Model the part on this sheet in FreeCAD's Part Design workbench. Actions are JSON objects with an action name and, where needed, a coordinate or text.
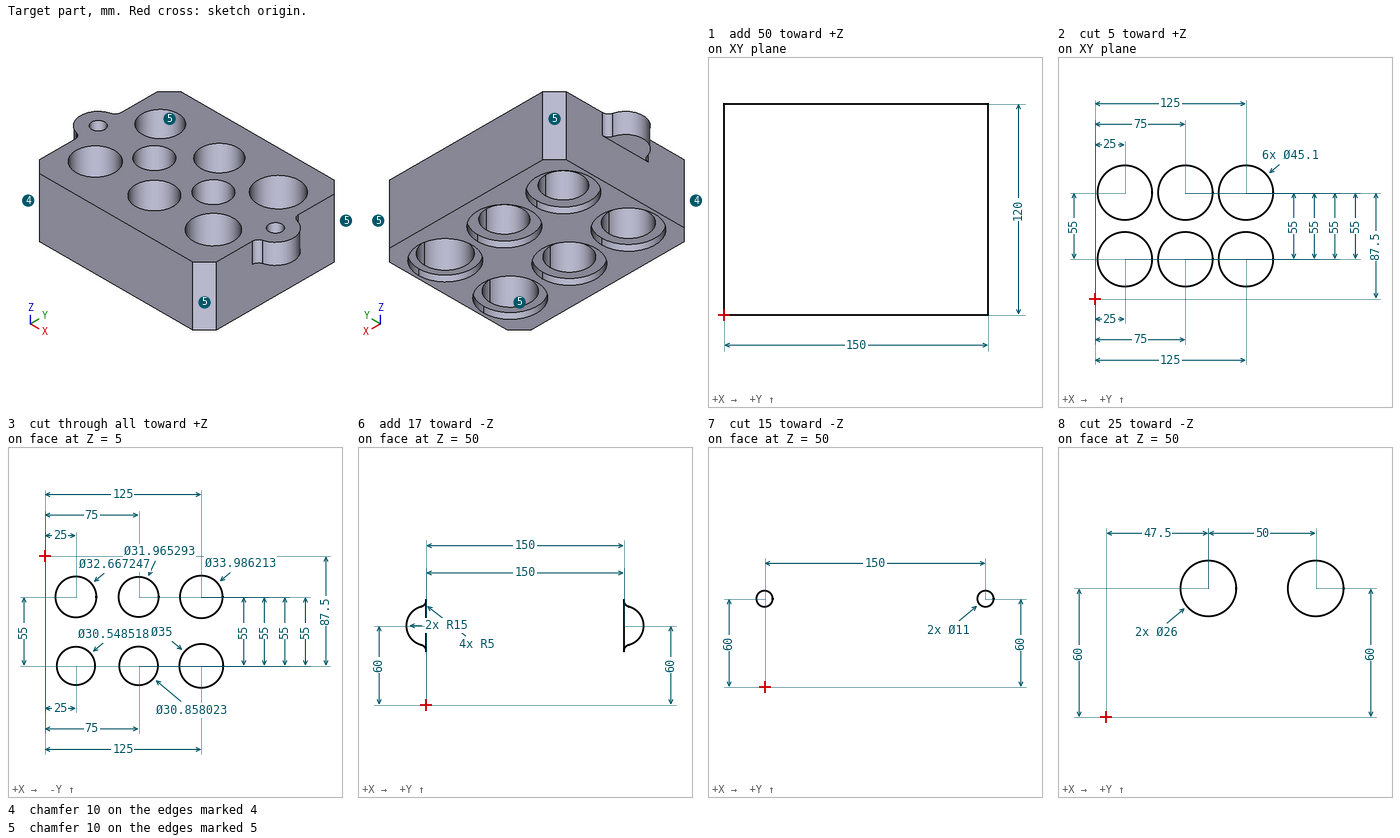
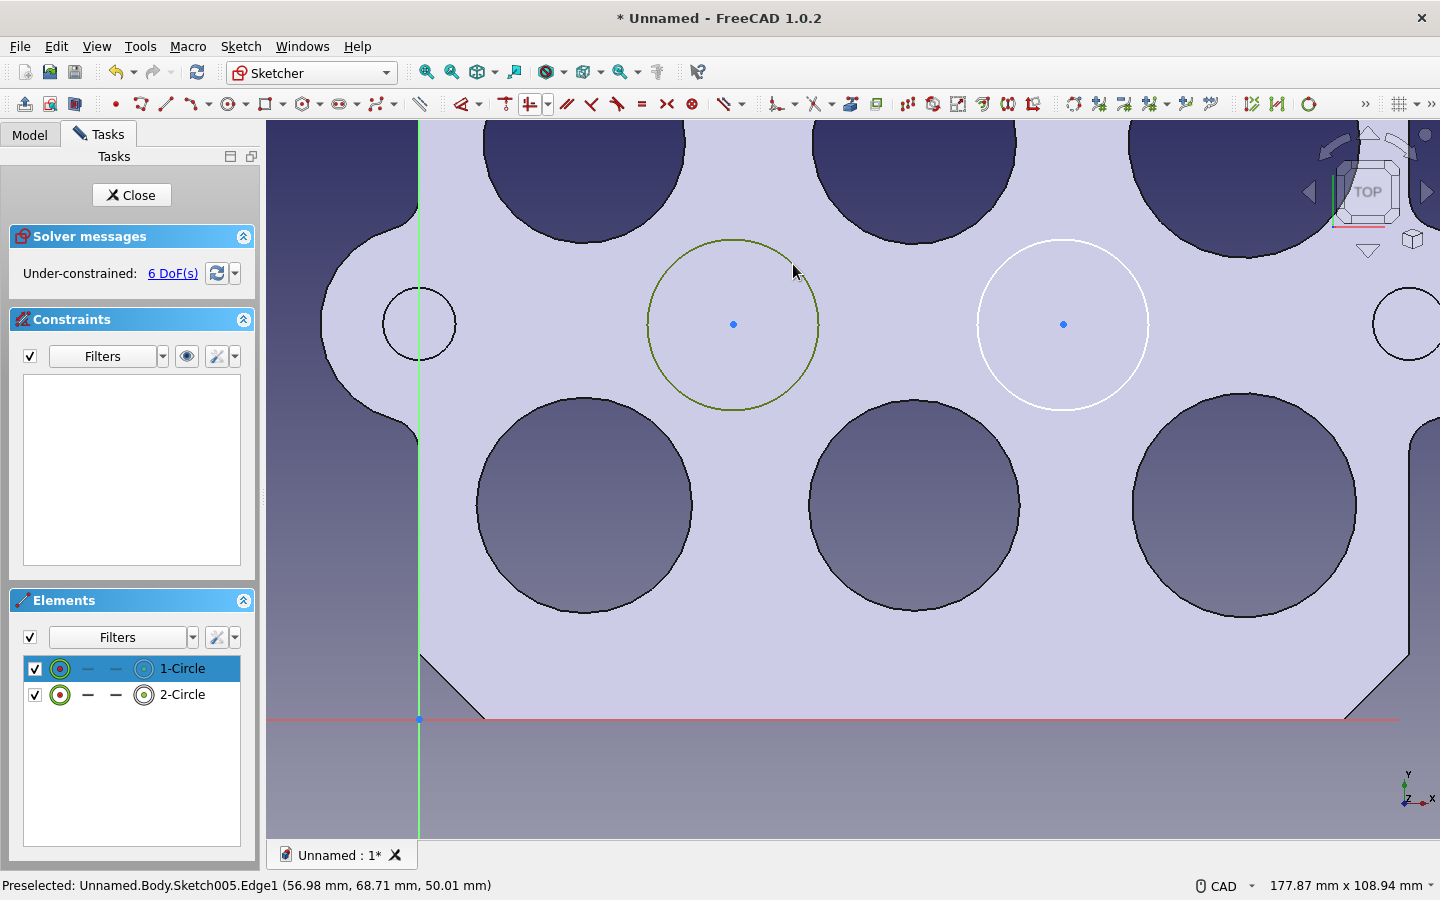
{"action": "left_click", "coordinate": [1123, 264]}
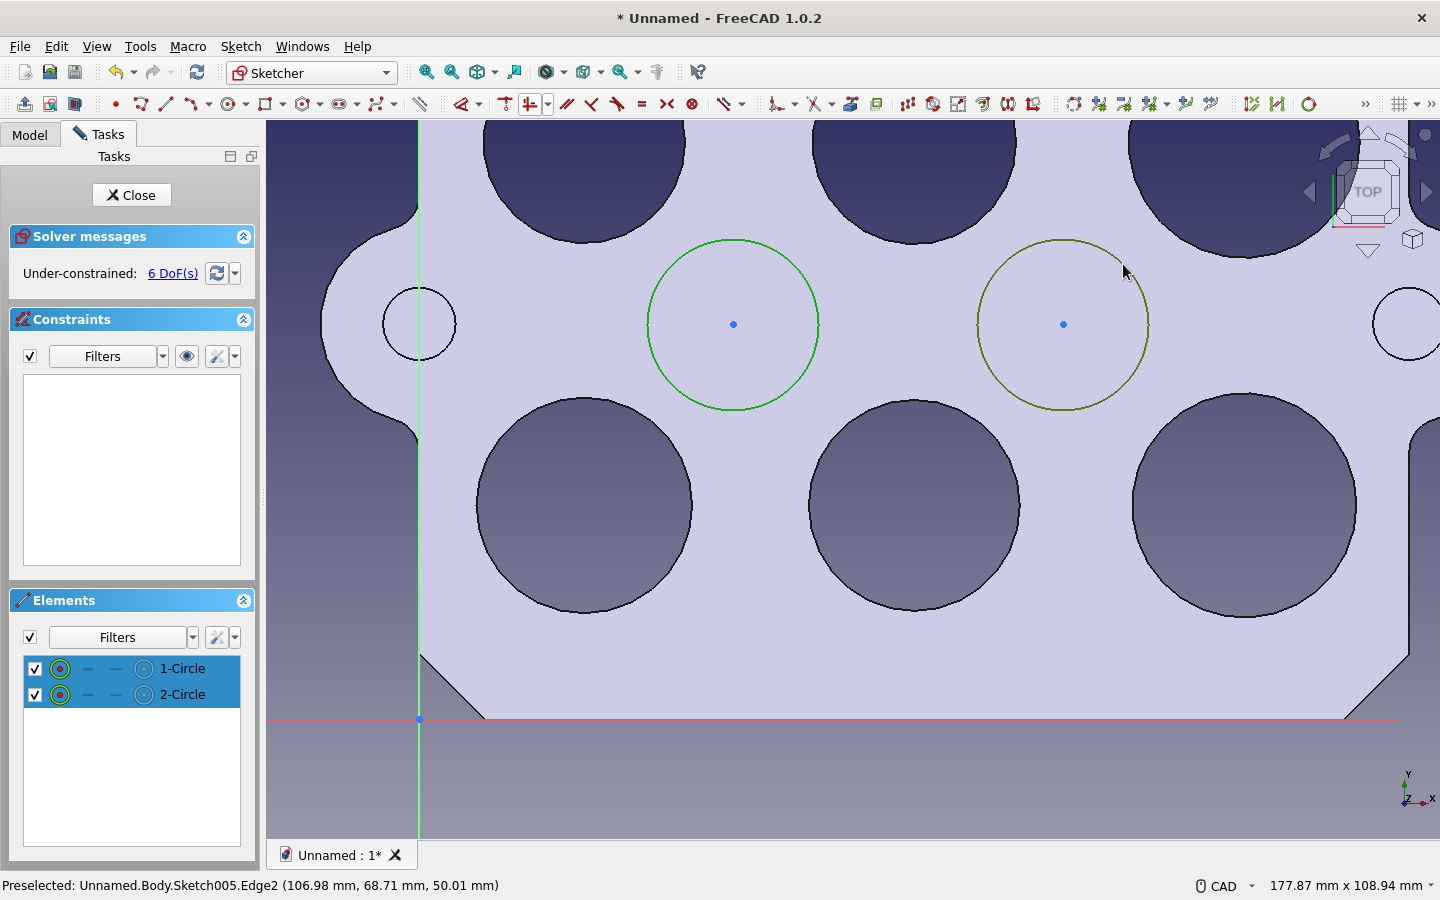
{"action": "left_click", "coordinate": [642, 104]}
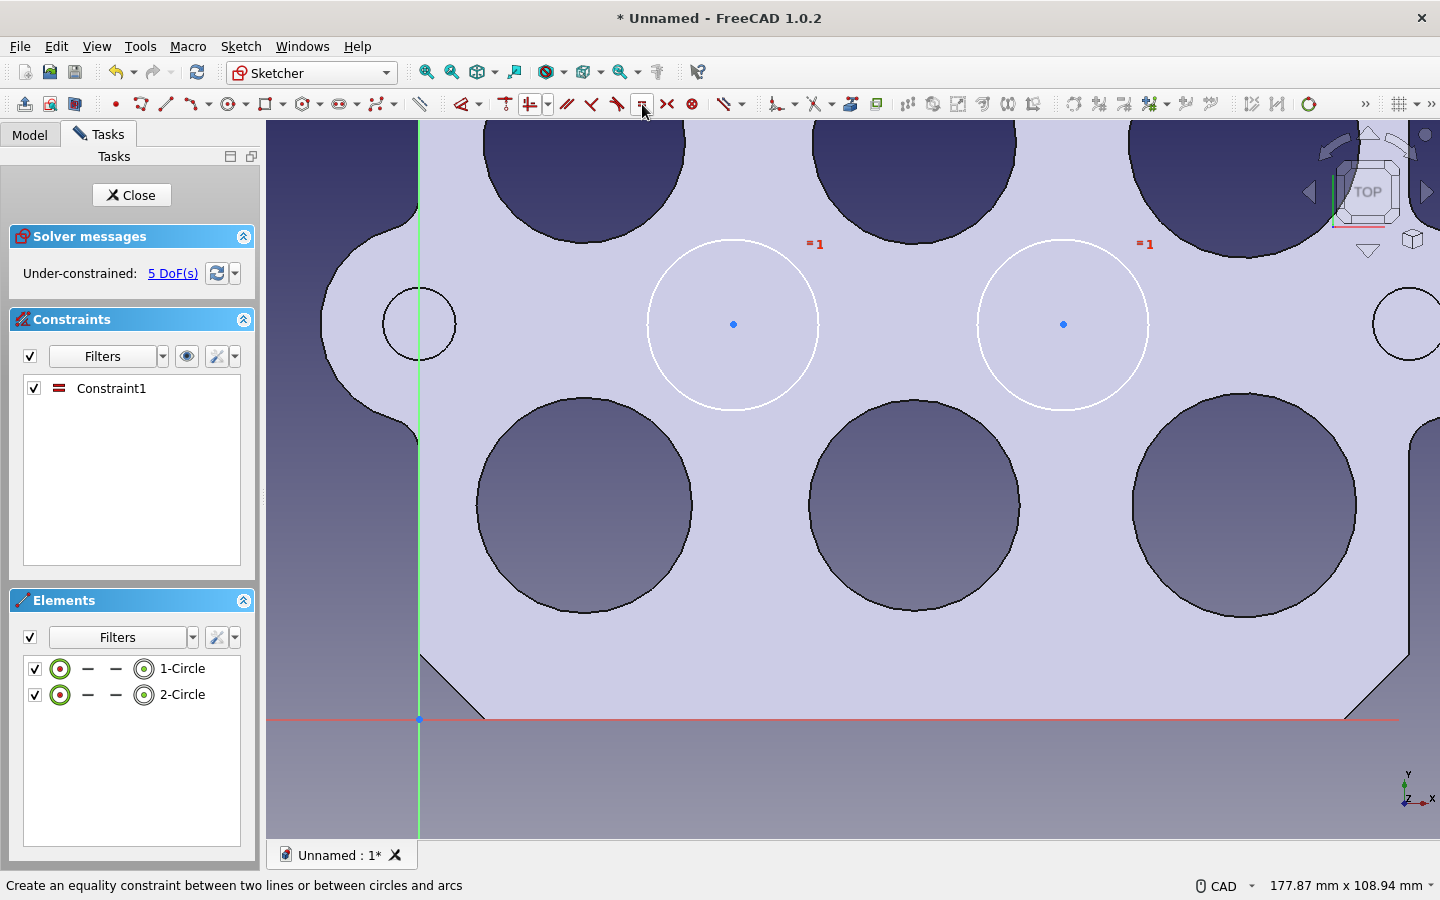
{"action": "left_click", "coordinate": [460, 104]}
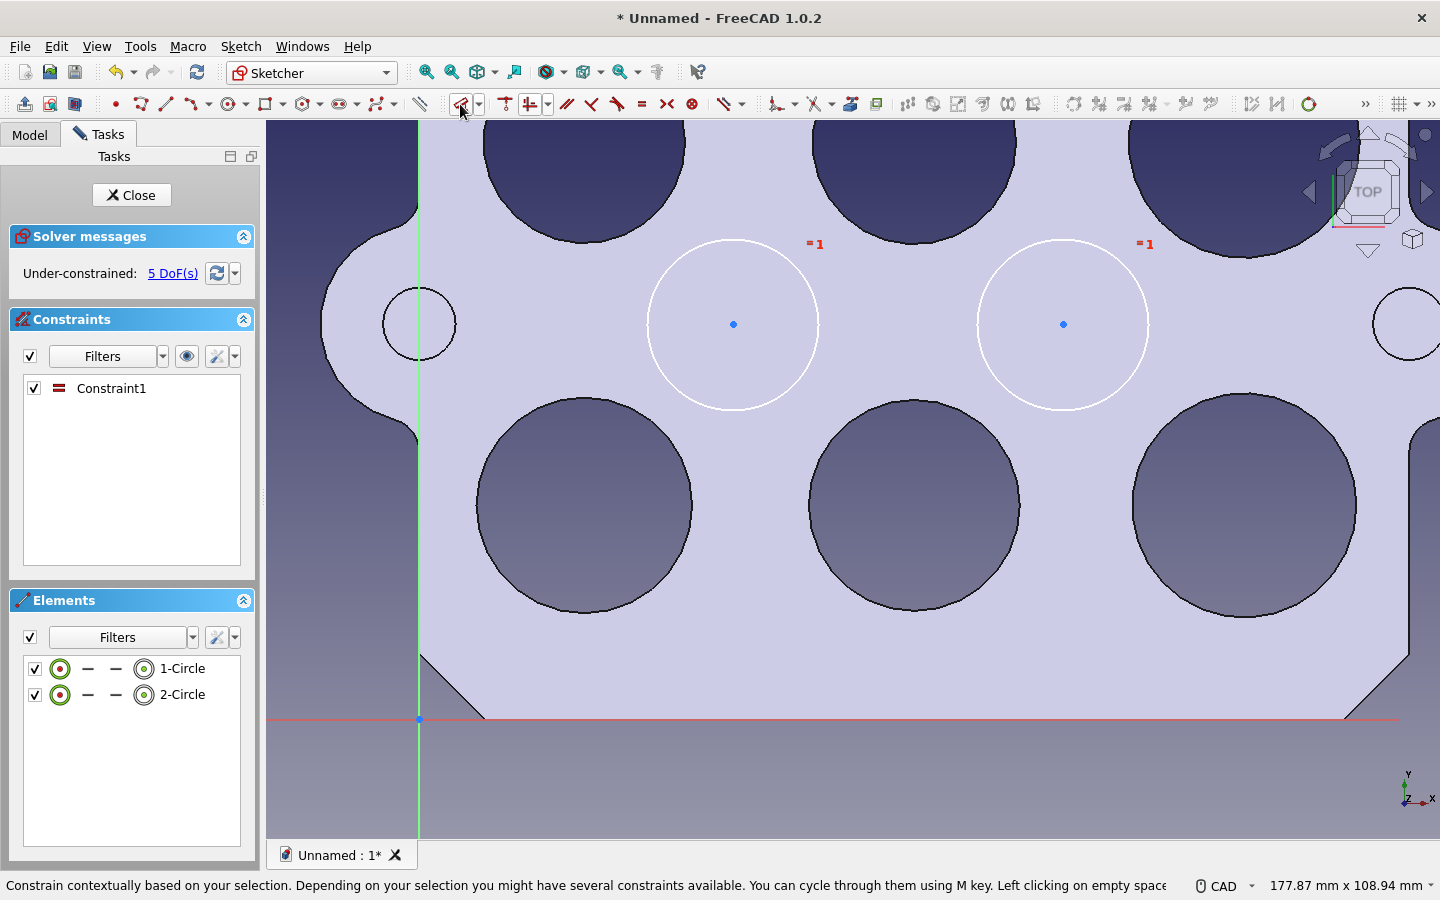
{"action": "left_click", "coordinate": [793, 264]}
{"action": "left_click", "coordinate": [815, 241]}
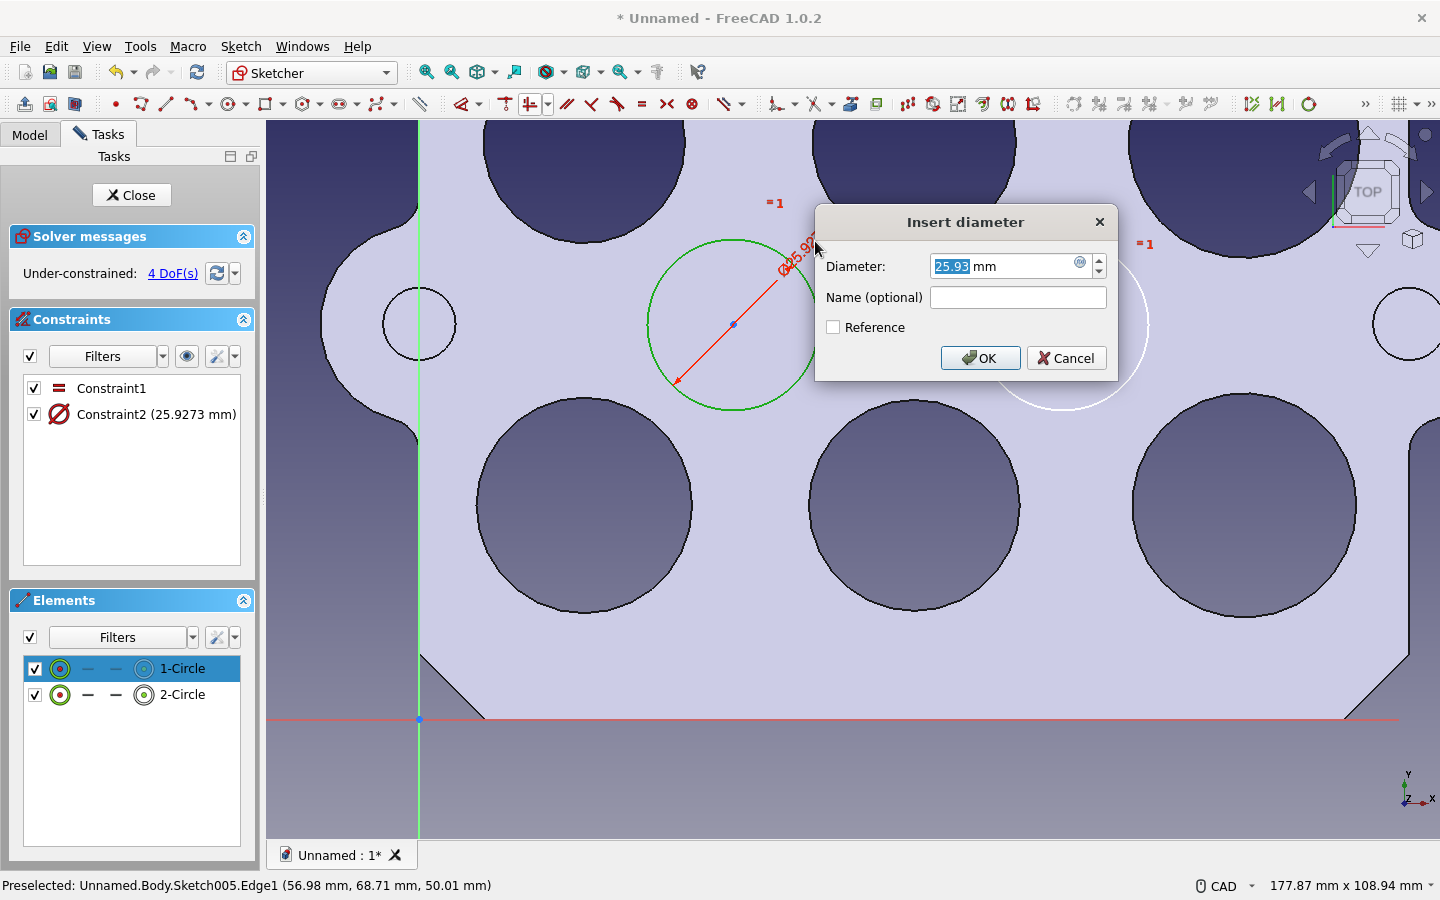
{"action": "type", "text": "26"}
{"action": "key", "text": "Return"}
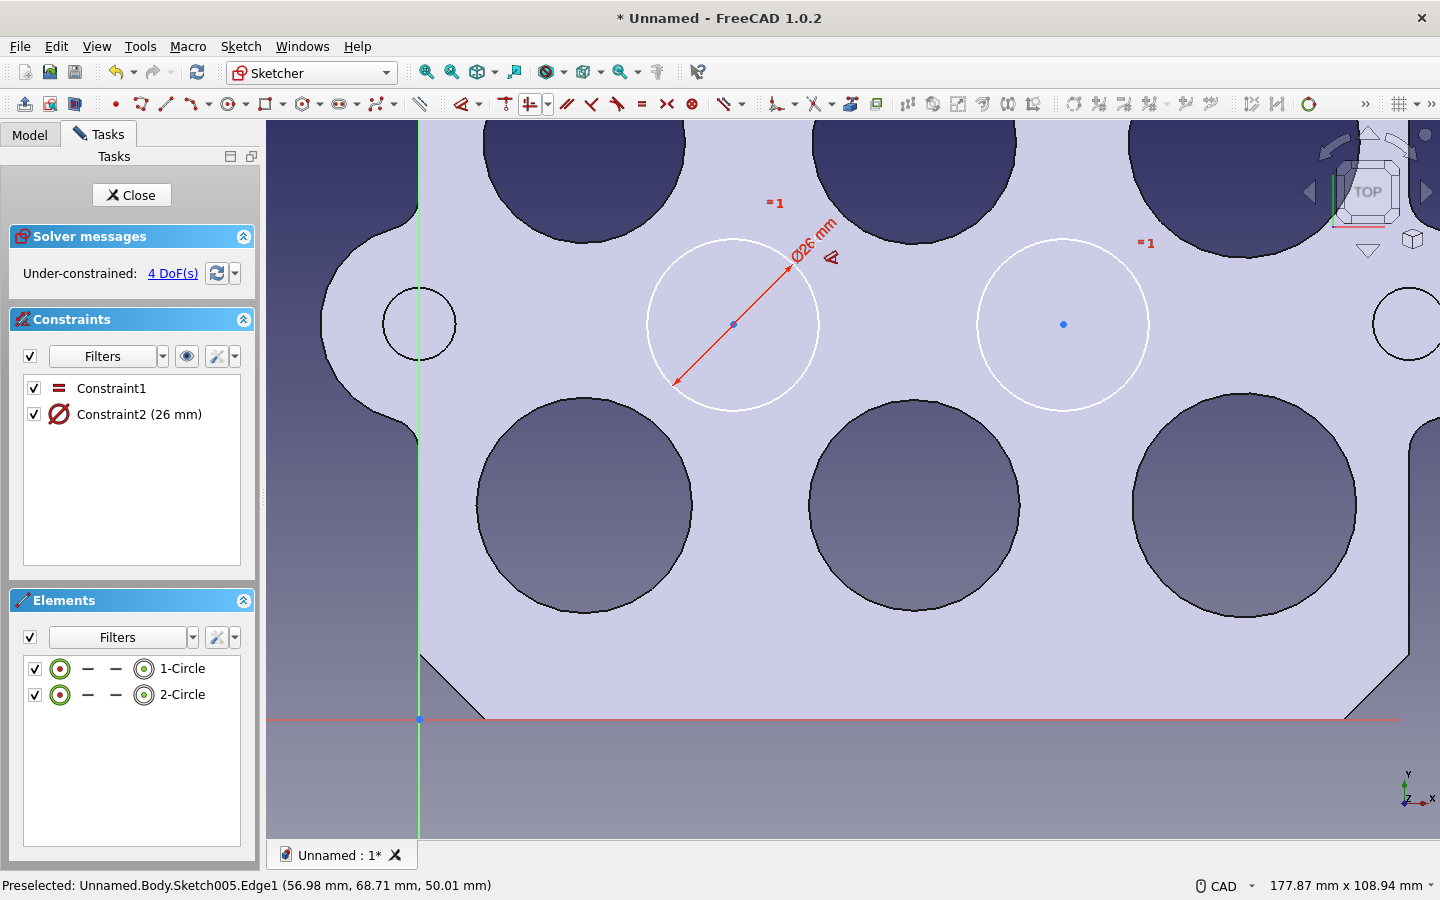
{"action": "left_click", "coordinate": [733, 325]}
{"action": "left_click", "coordinate": [385, 522]}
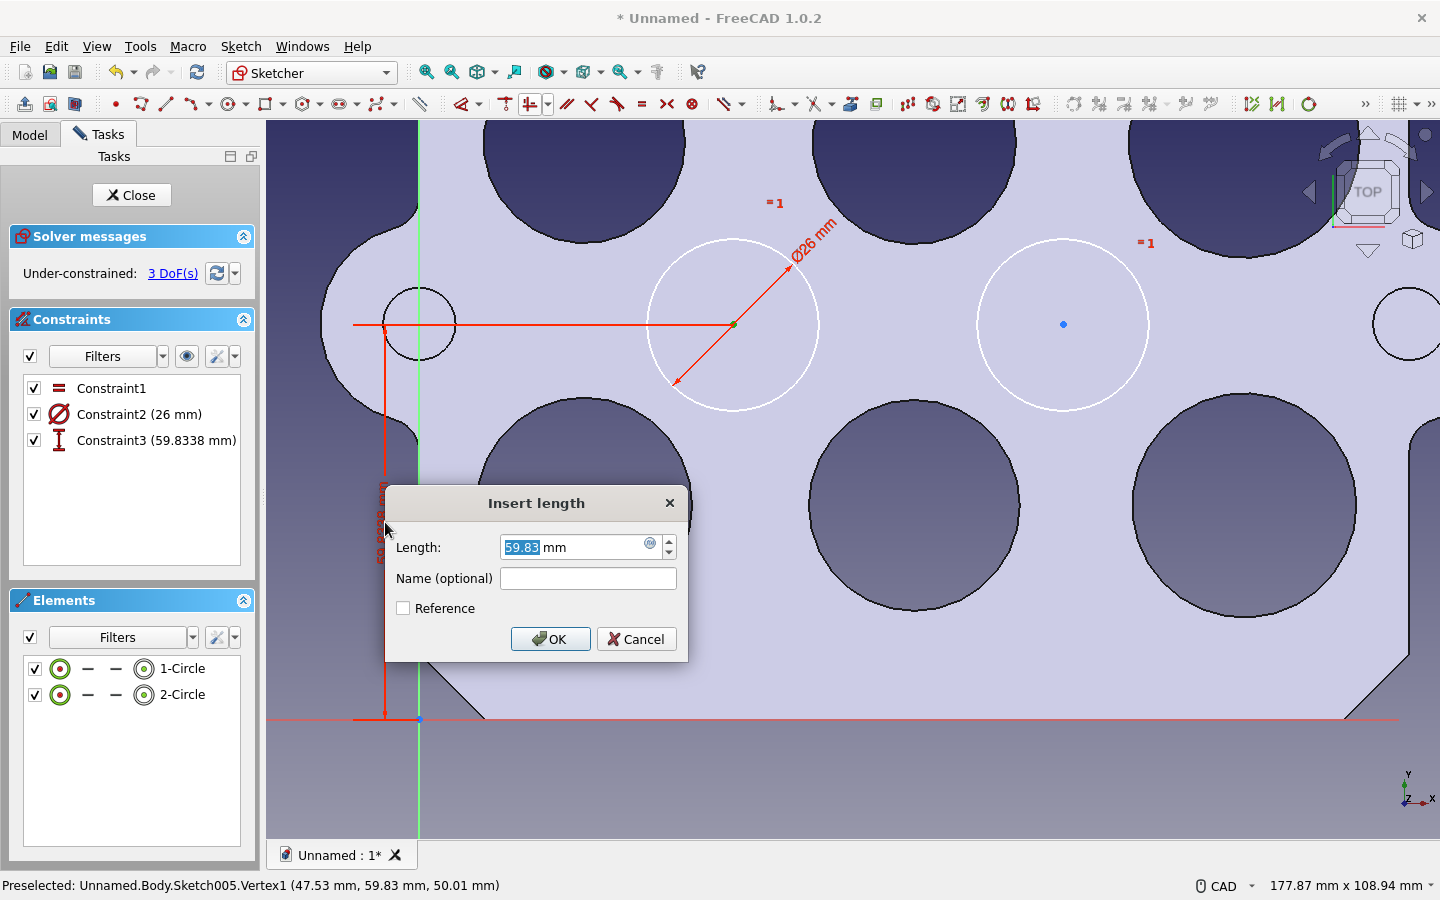
{"action": "type", "text": "60"}
{"action": "key", "text": "Return"}